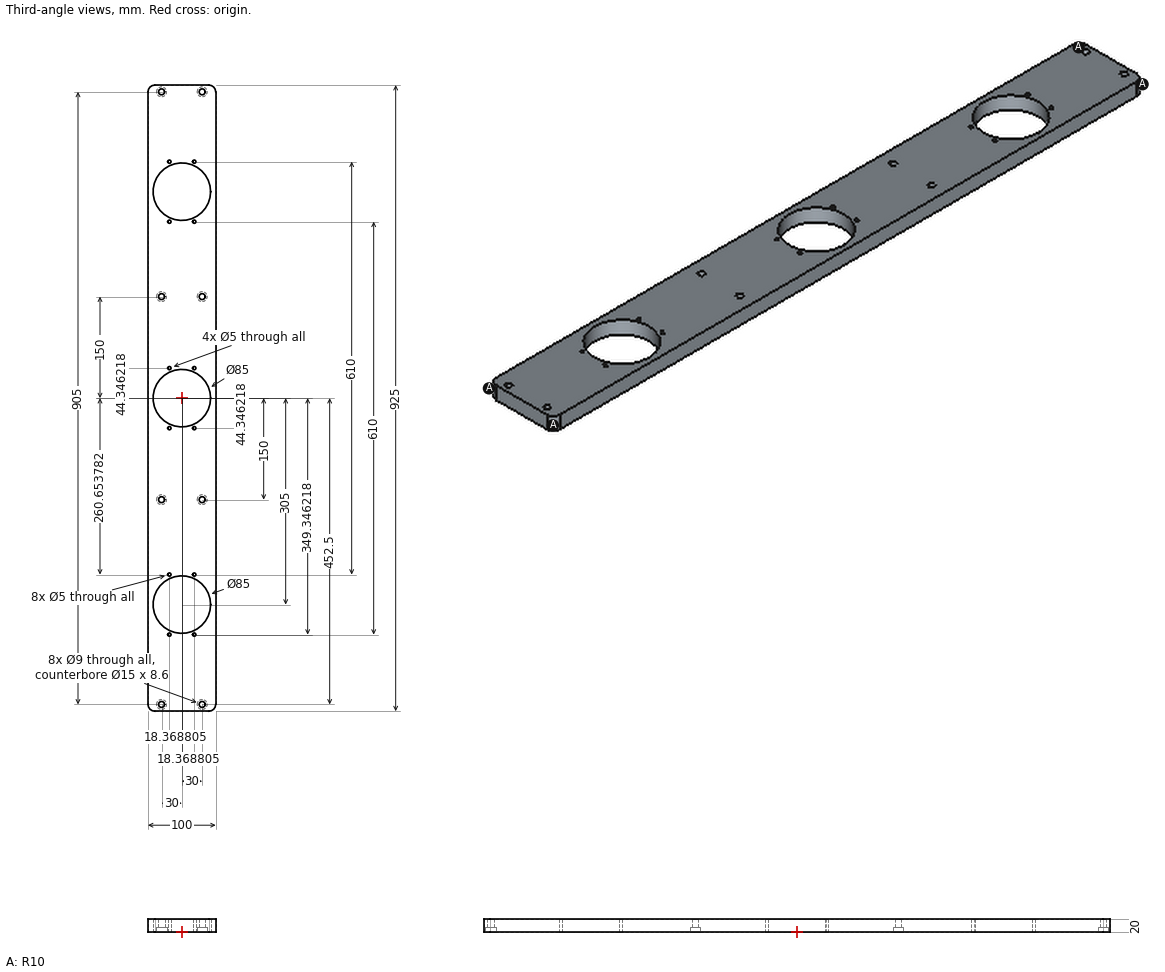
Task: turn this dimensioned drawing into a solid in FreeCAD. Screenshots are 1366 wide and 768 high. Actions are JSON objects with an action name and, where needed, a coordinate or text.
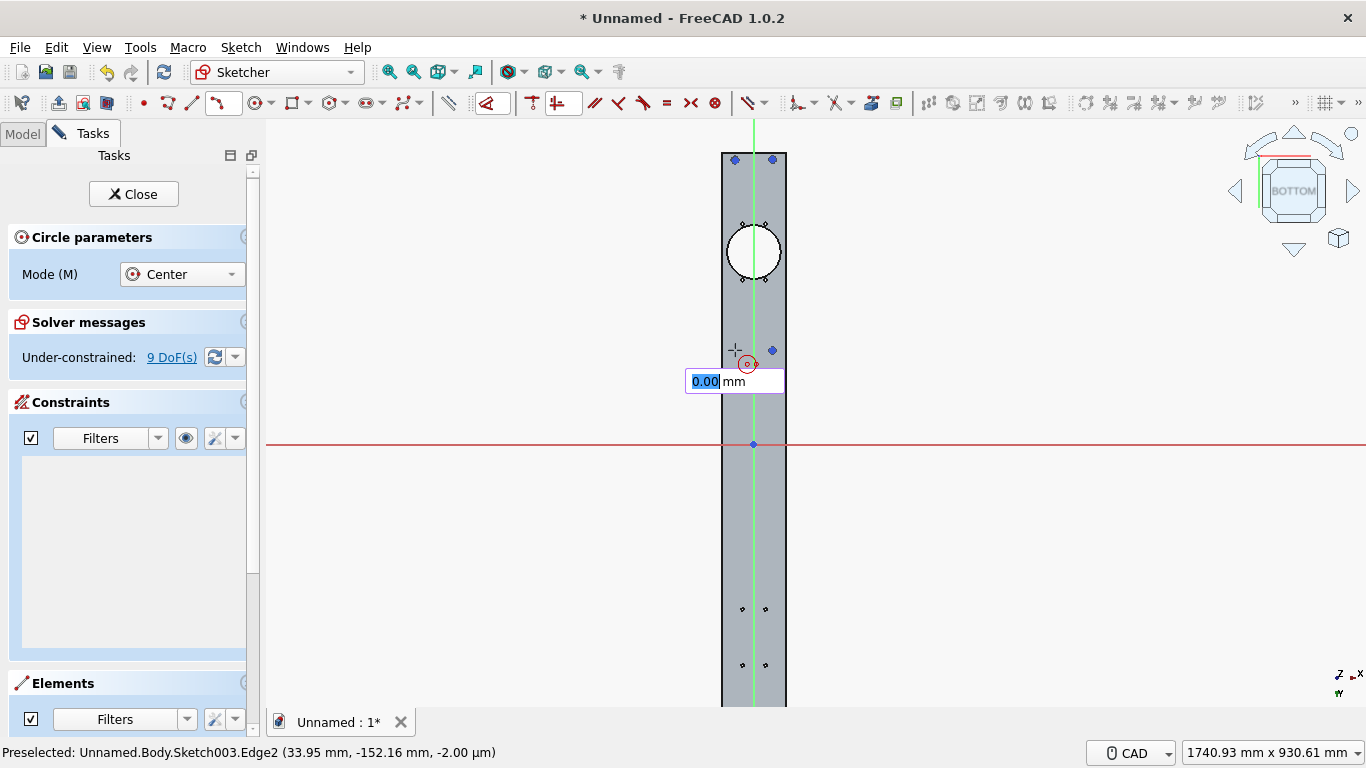
{"action": "scroll", "coordinate": [737, 348], "scroll_direction": "up", "scroll_amount": 9}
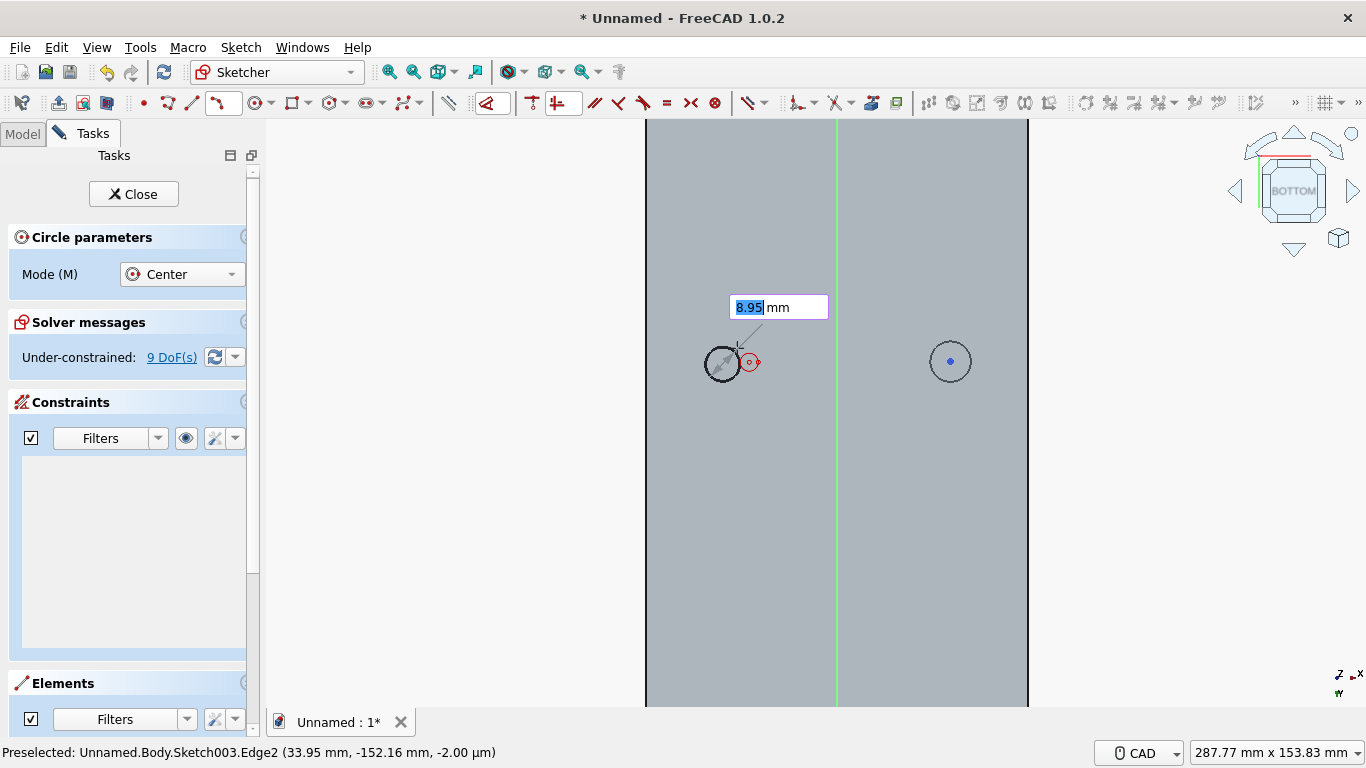
{"action": "left_click", "coordinate": [735, 346]}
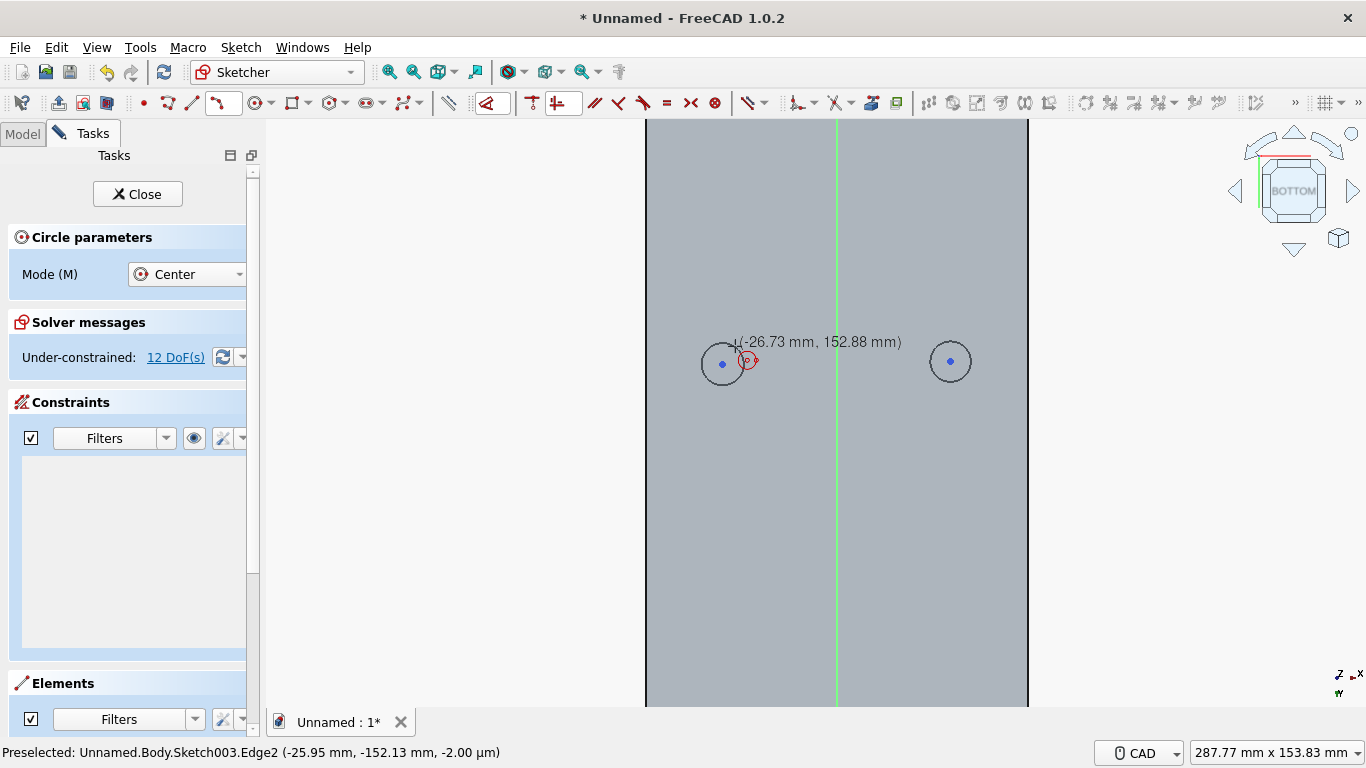
{"action": "scroll", "coordinate": [736, 348], "scroll_direction": "down", "scroll_amount": 11}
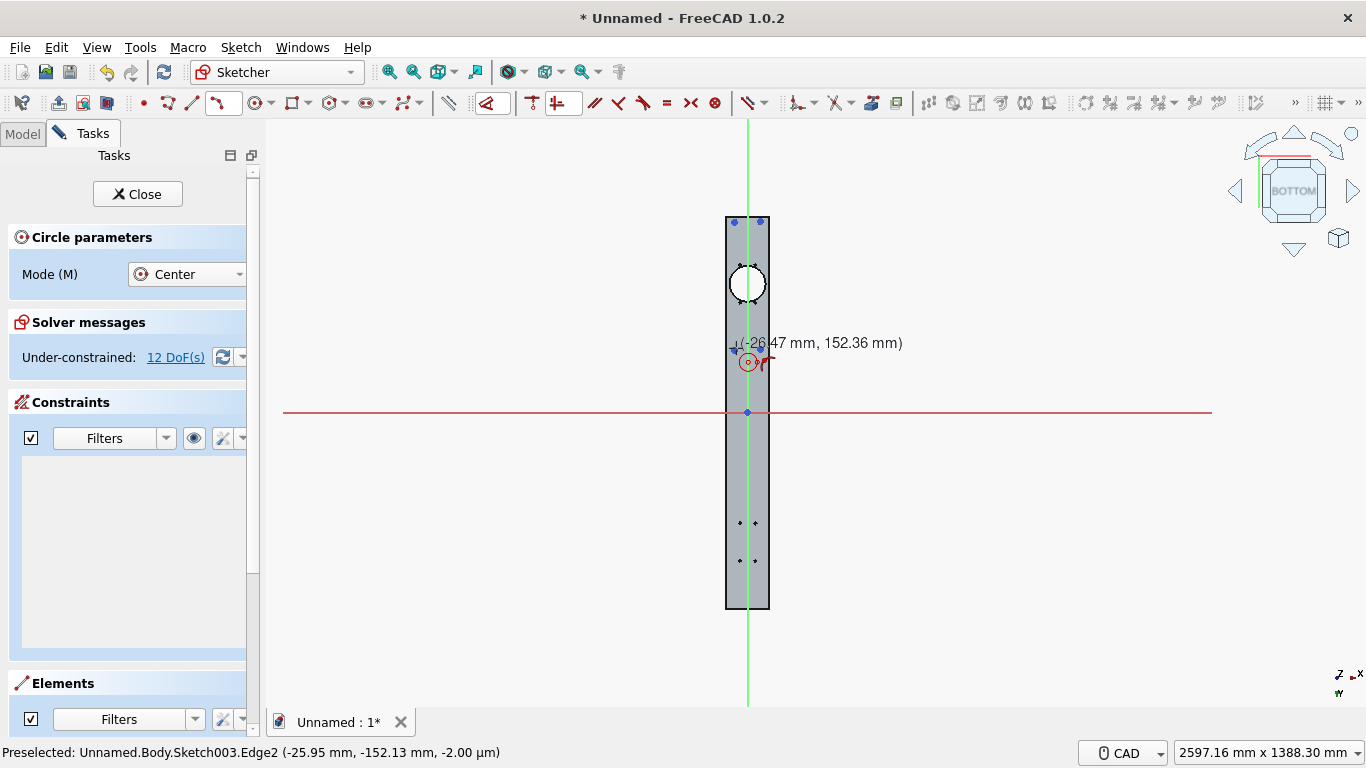
{"action": "scroll", "coordinate": [735, 477], "scroll_direction": "up", "scroll_amount": 13}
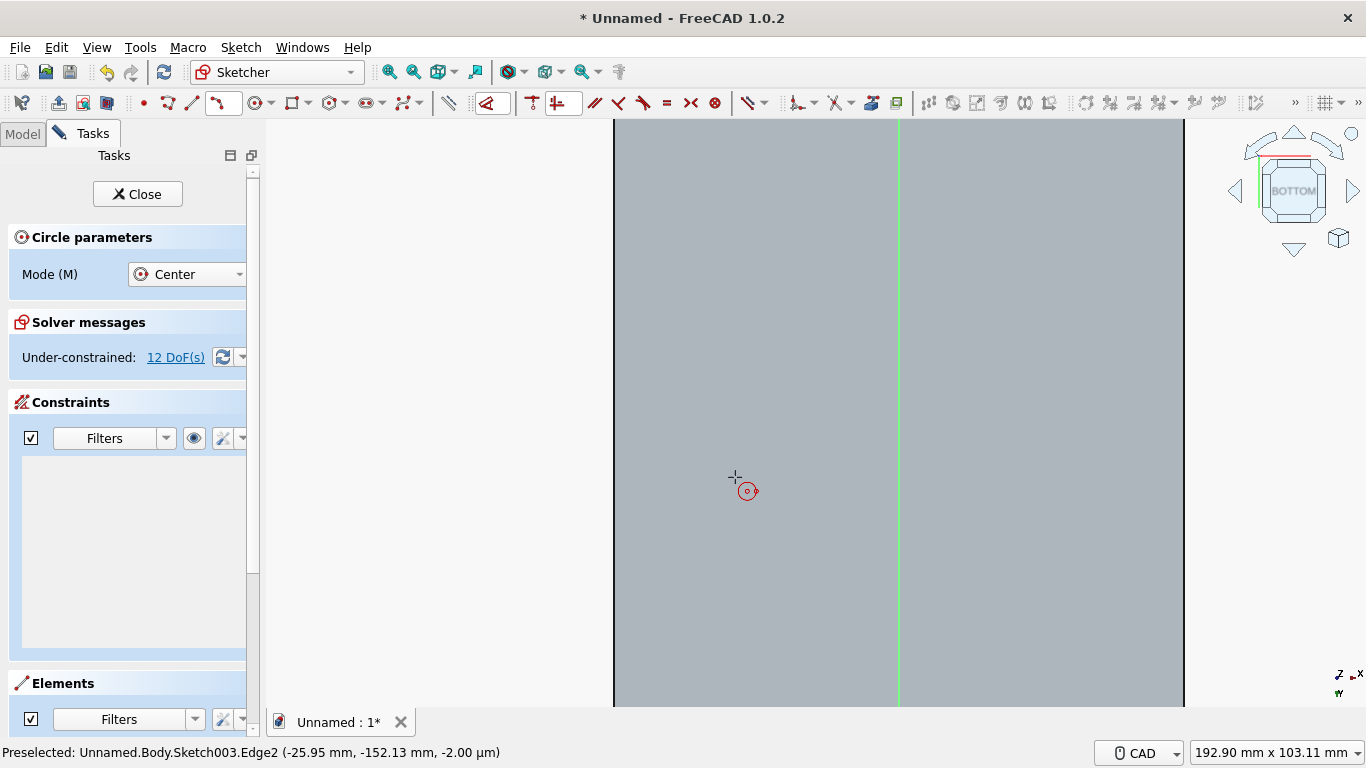
{"action": "scroll", "coordinate": [735, 478], "scroll_direction": "down", "scroll_amount": 13}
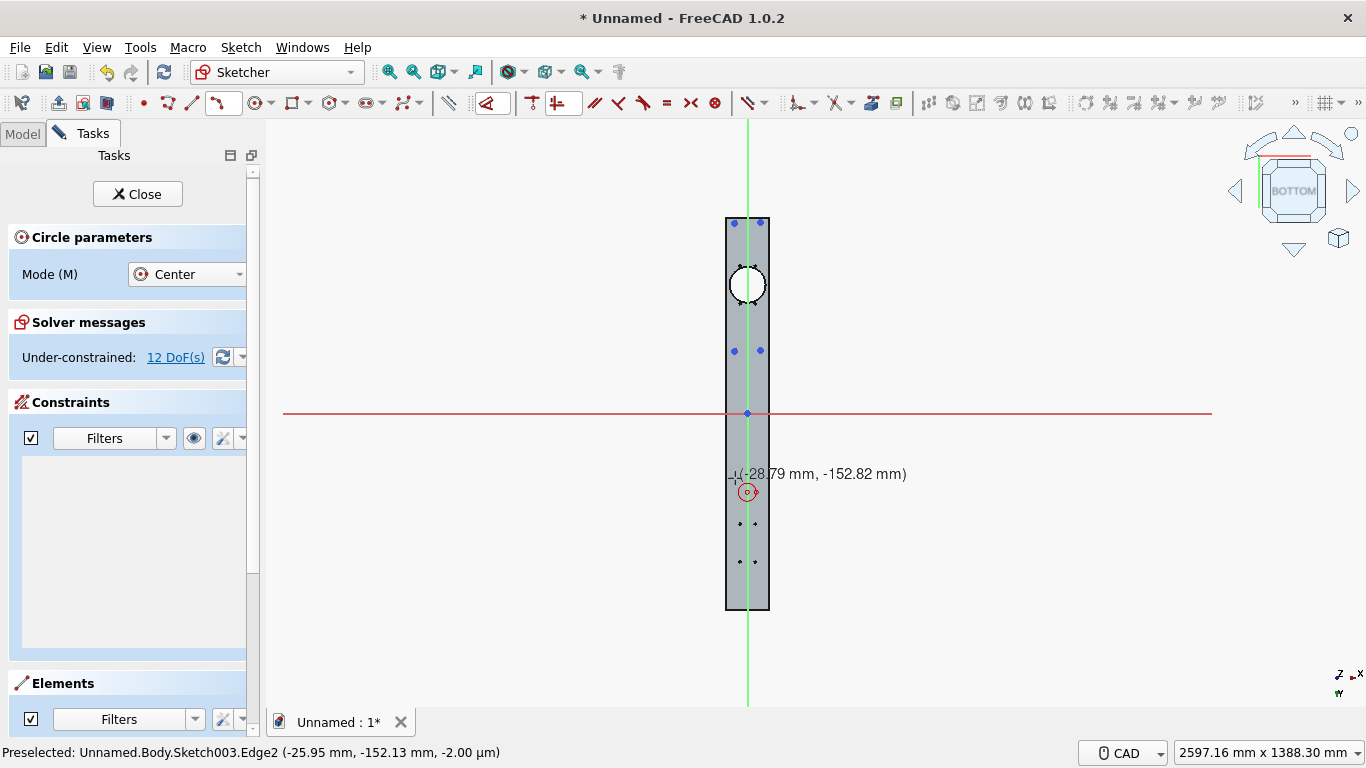
{"action": "scroll", "coordinate": [735, 477], "scroll_direction": "up", "scroll_amount": 2}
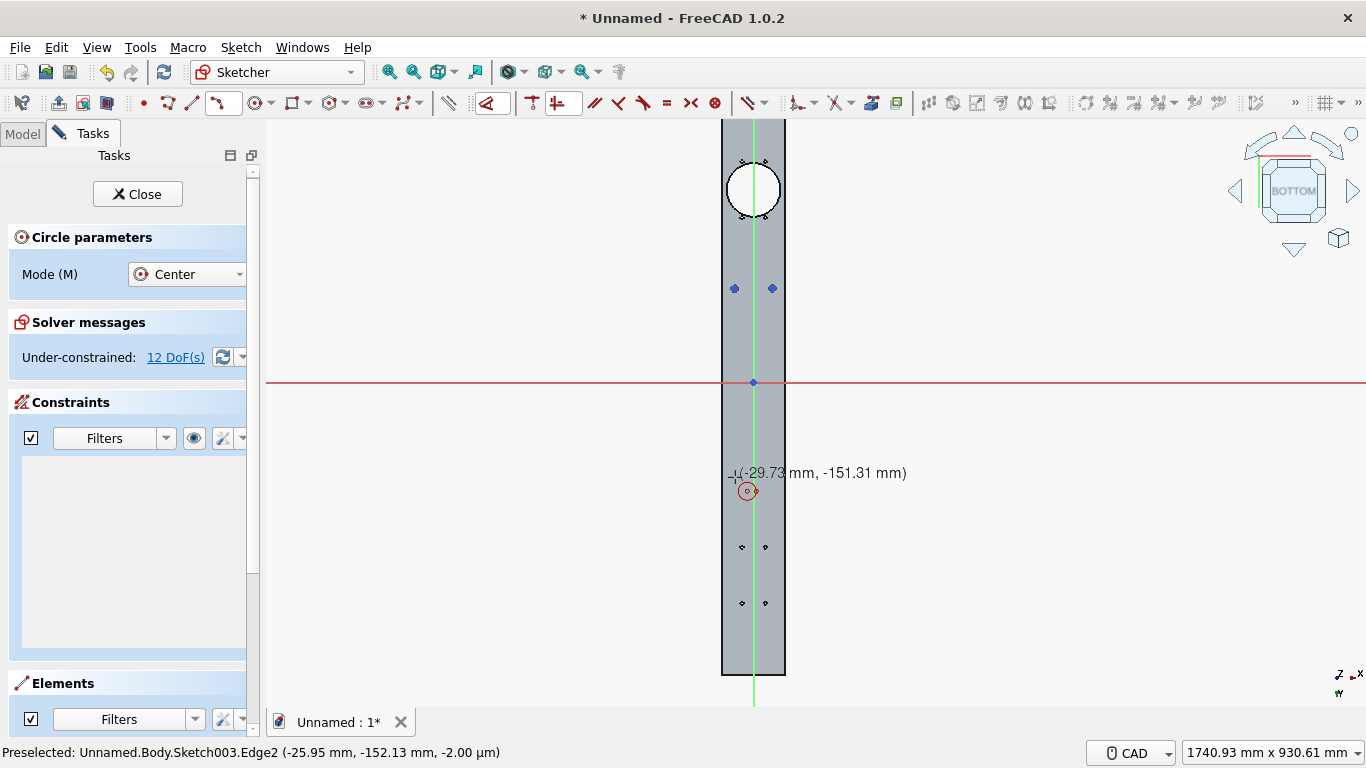
{"action": "left_click", "coordinate": [735, 477]}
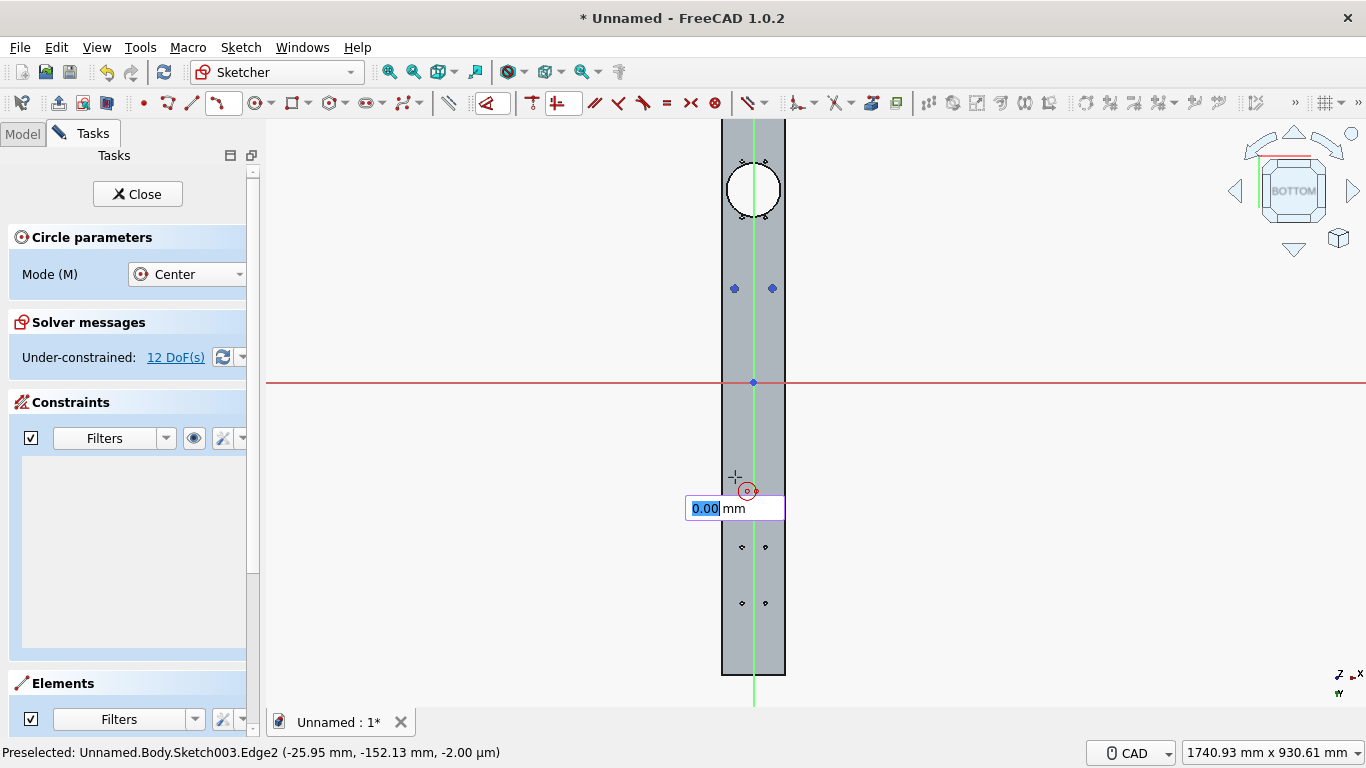
{"action": "scroll", "coordinate": [737, 475], "scroll_direction": "up", "scroll_amount": 9}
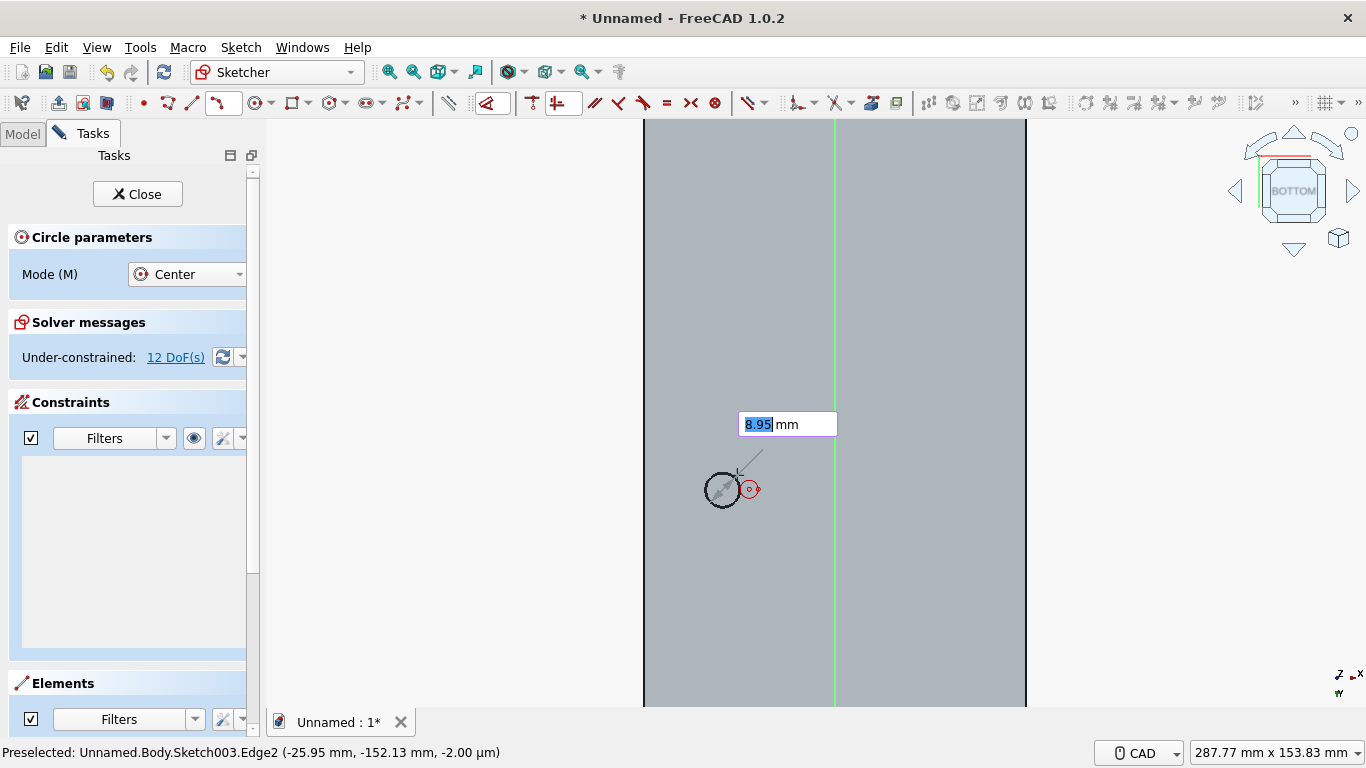
{"action": "left_click", "coordinate": [733, 474]}